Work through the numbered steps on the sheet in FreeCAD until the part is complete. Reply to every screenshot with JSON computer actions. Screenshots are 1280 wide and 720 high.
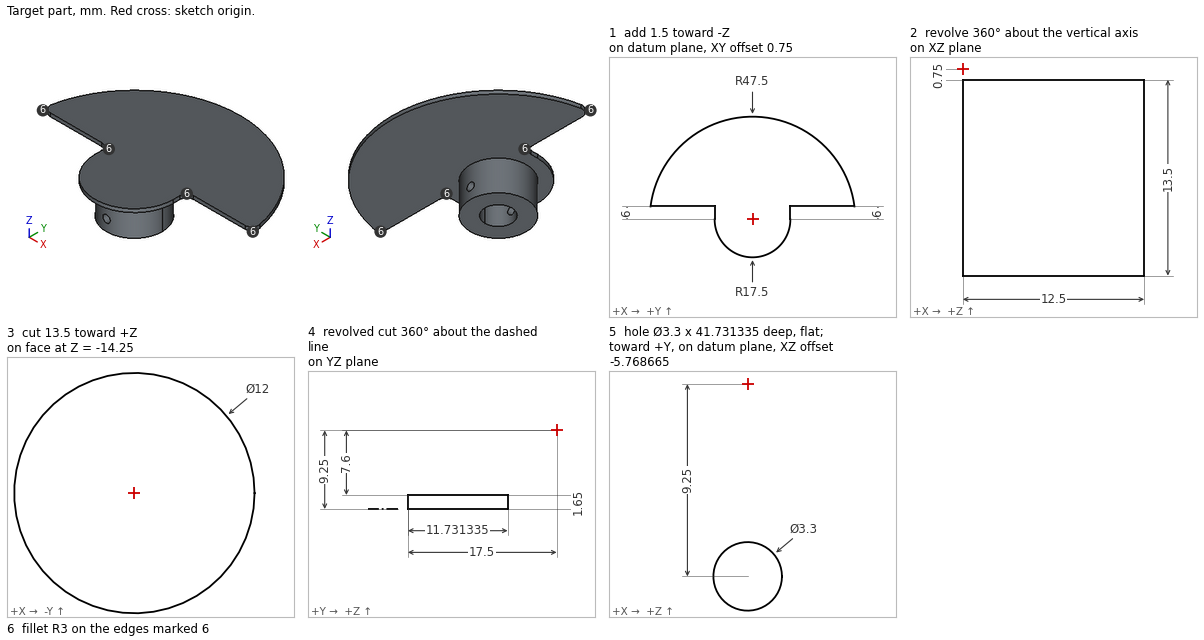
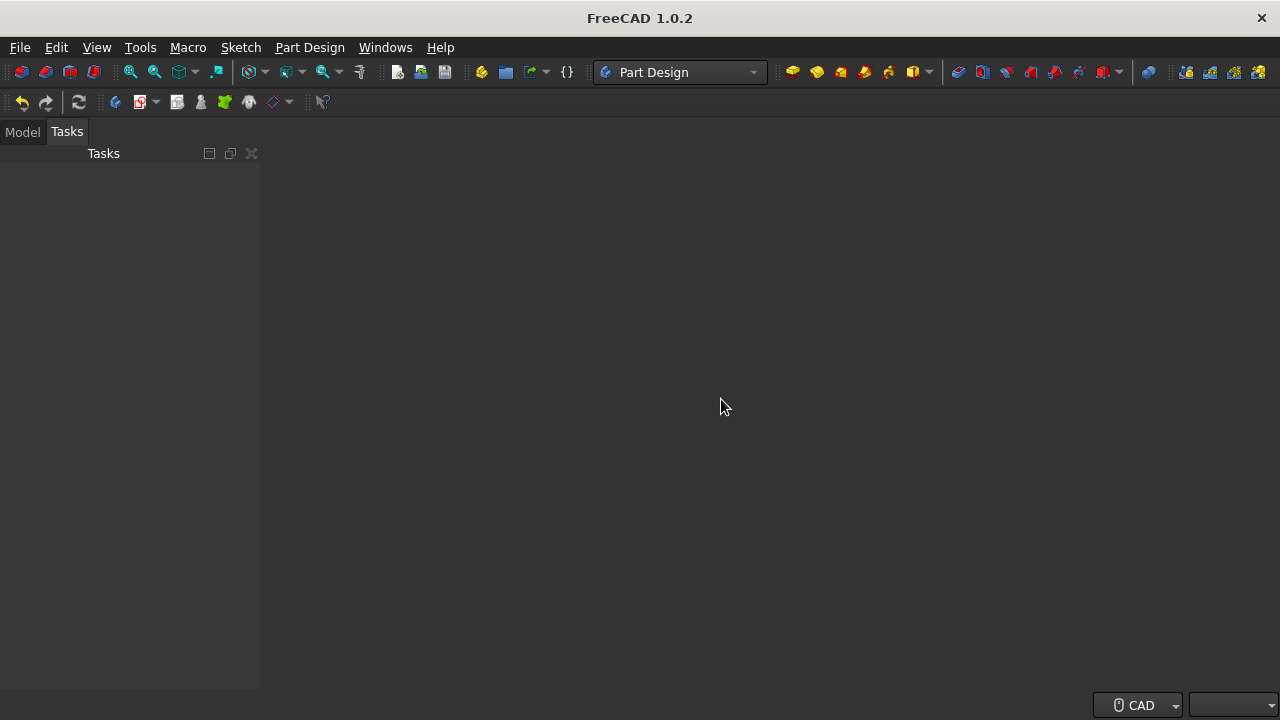
{"action": "left_click", "coordinate": [398, 72]}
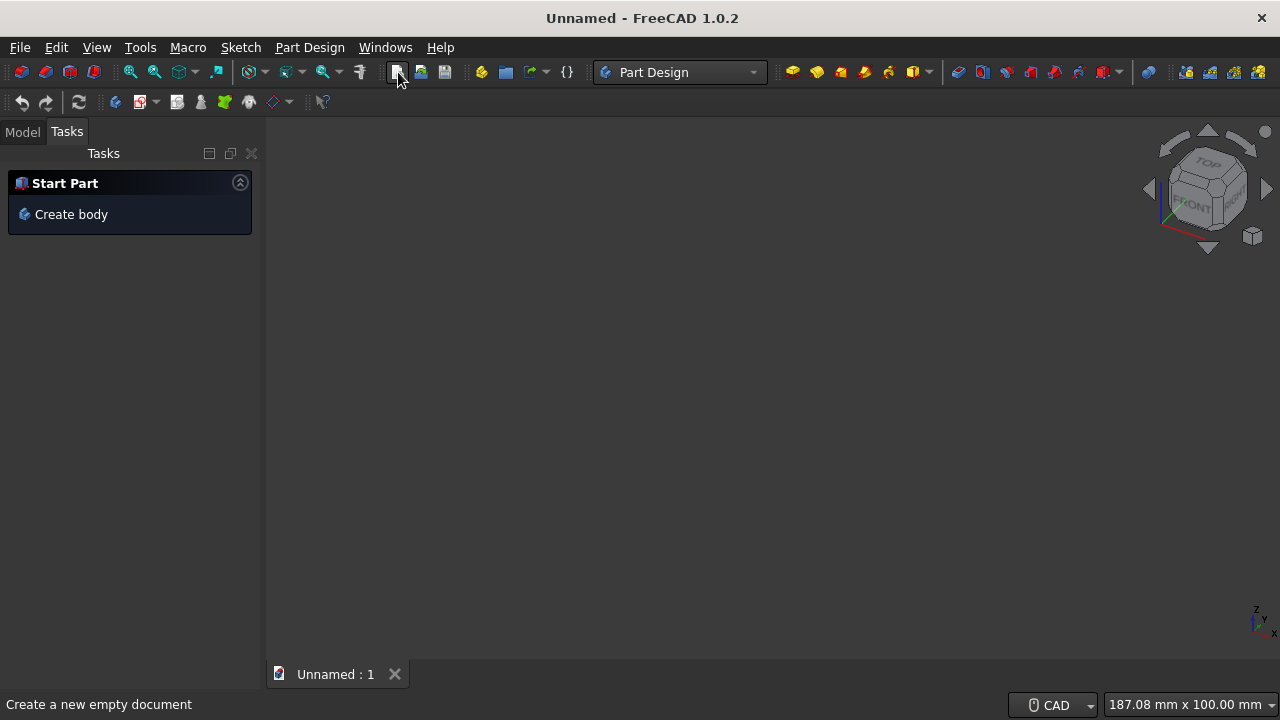
{"action": "left_click", "coordinate": [116, 102]}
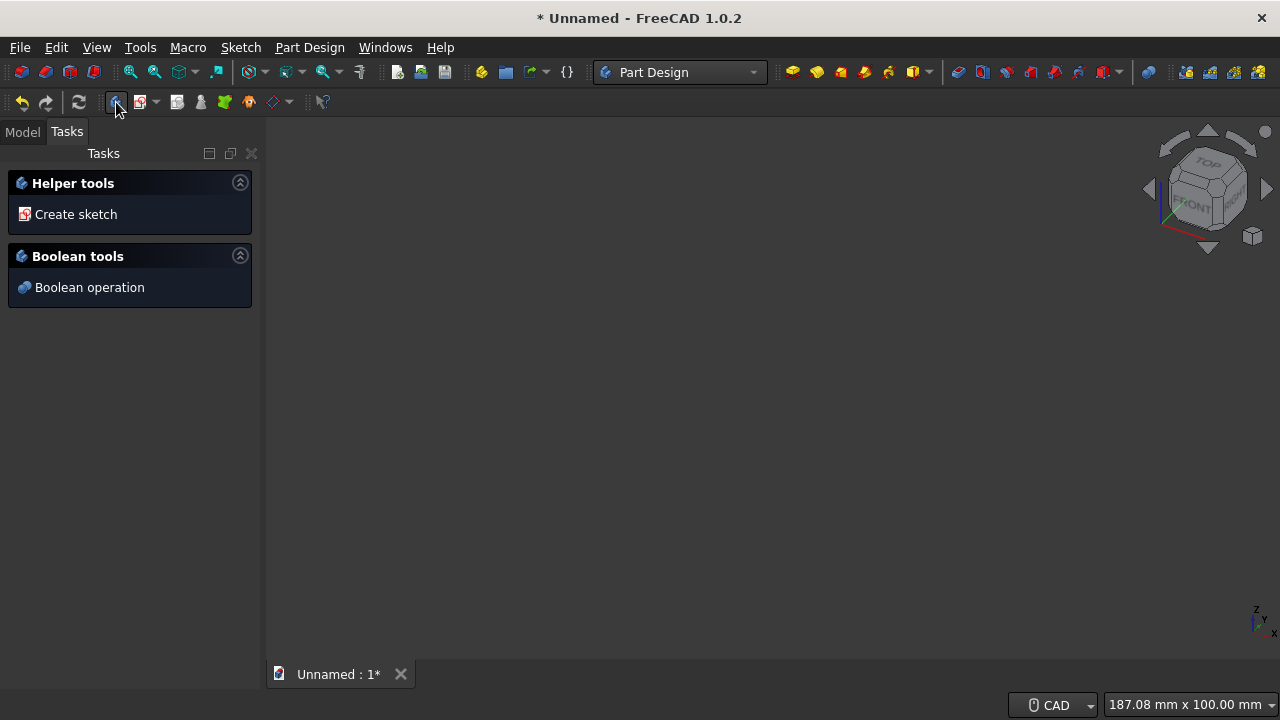
{"action": "left_click", "coordinate": [23, 131]}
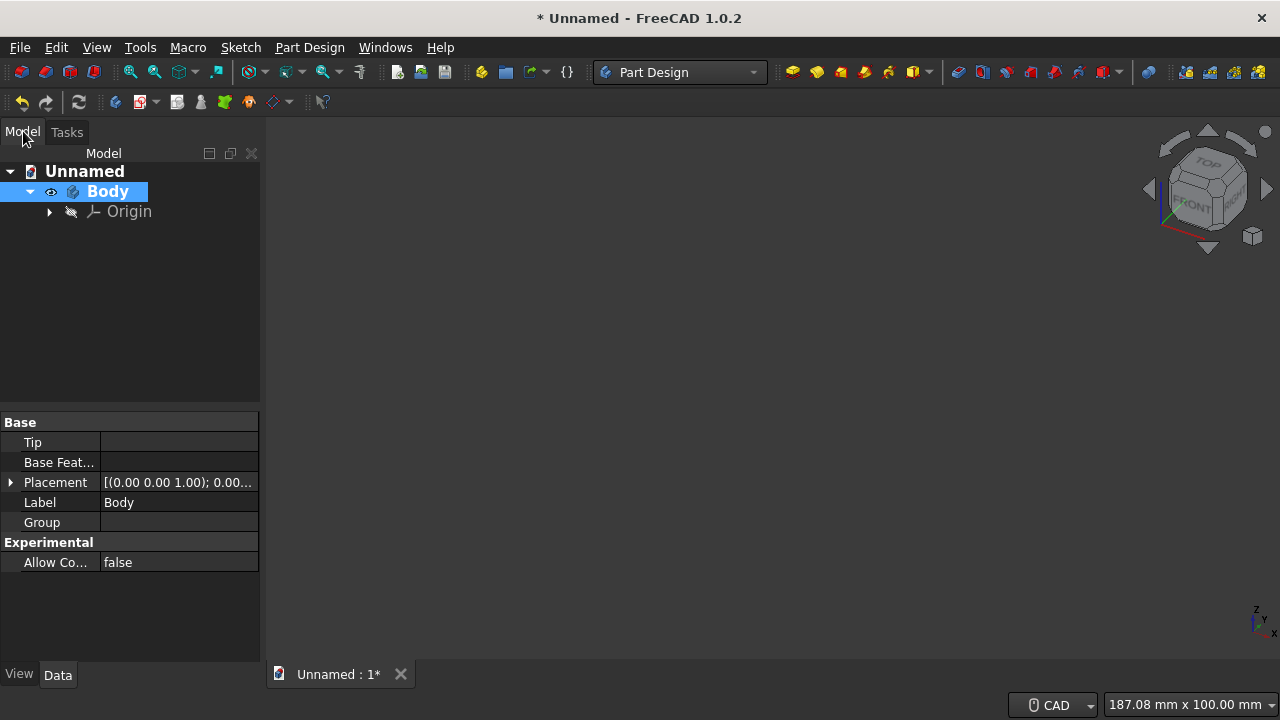
{"action": "left_click", "coordinate": [50, 212]}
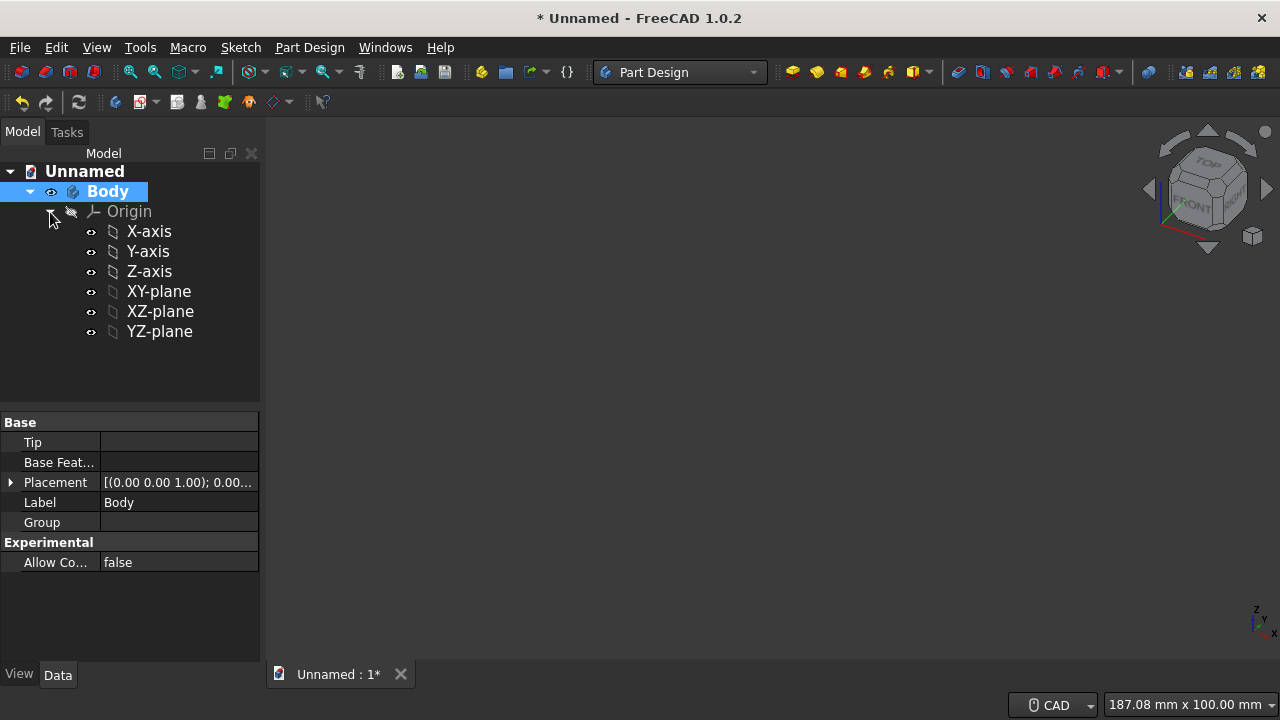
{"action": "left_click", "coordinate": [136, 292]}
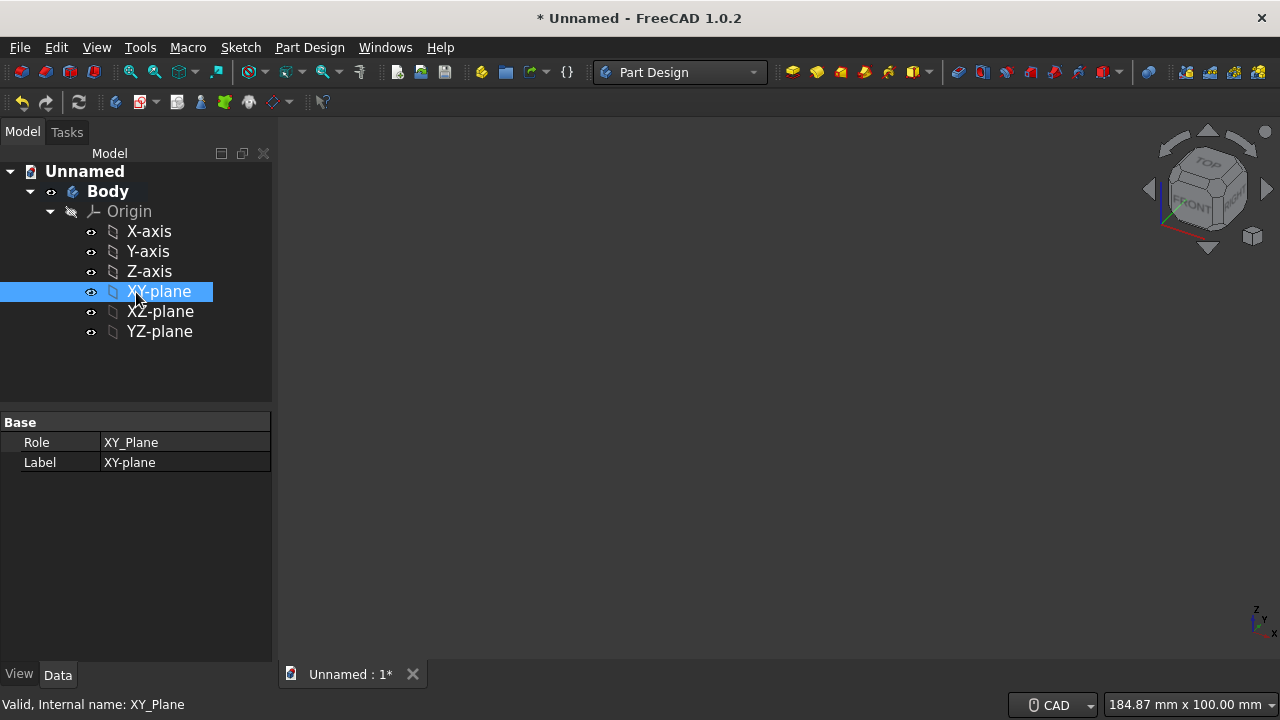
{"action": "left_click", "coordinate": [274, 102]}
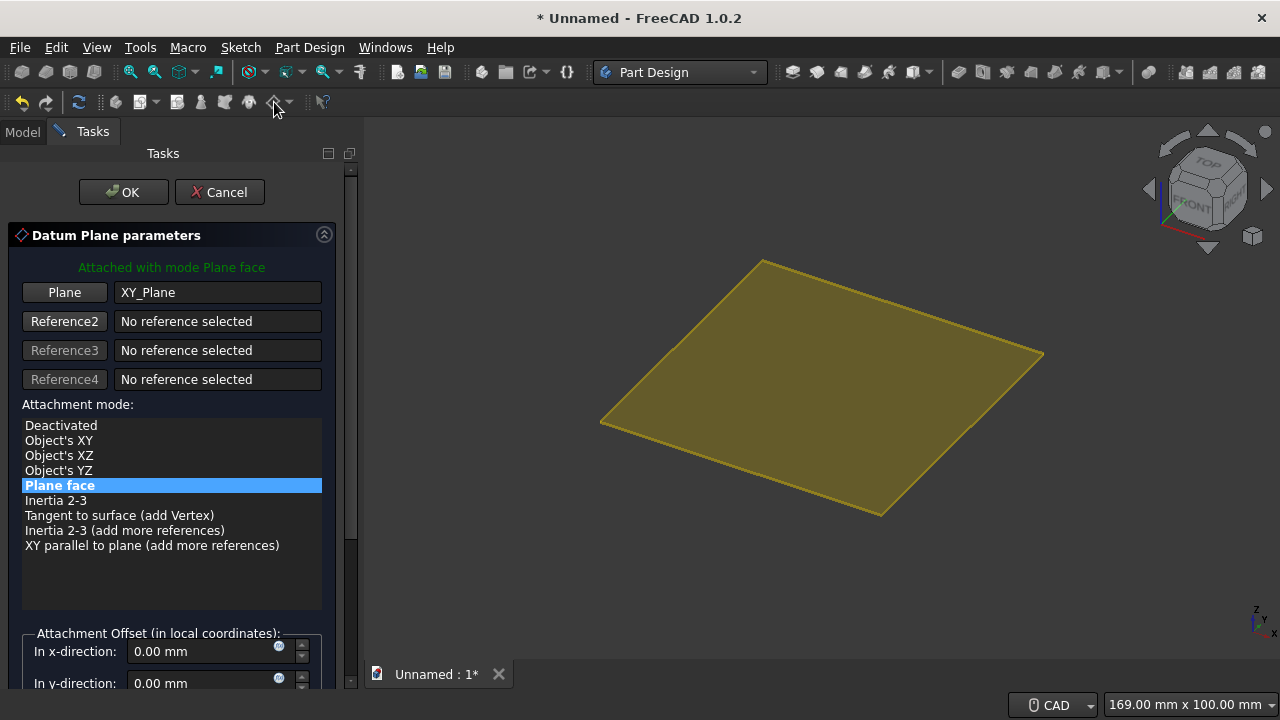
{"action": "scroll", "coordinate": [351, 426], "scroll_direction": "down", "scroll_amount": 2}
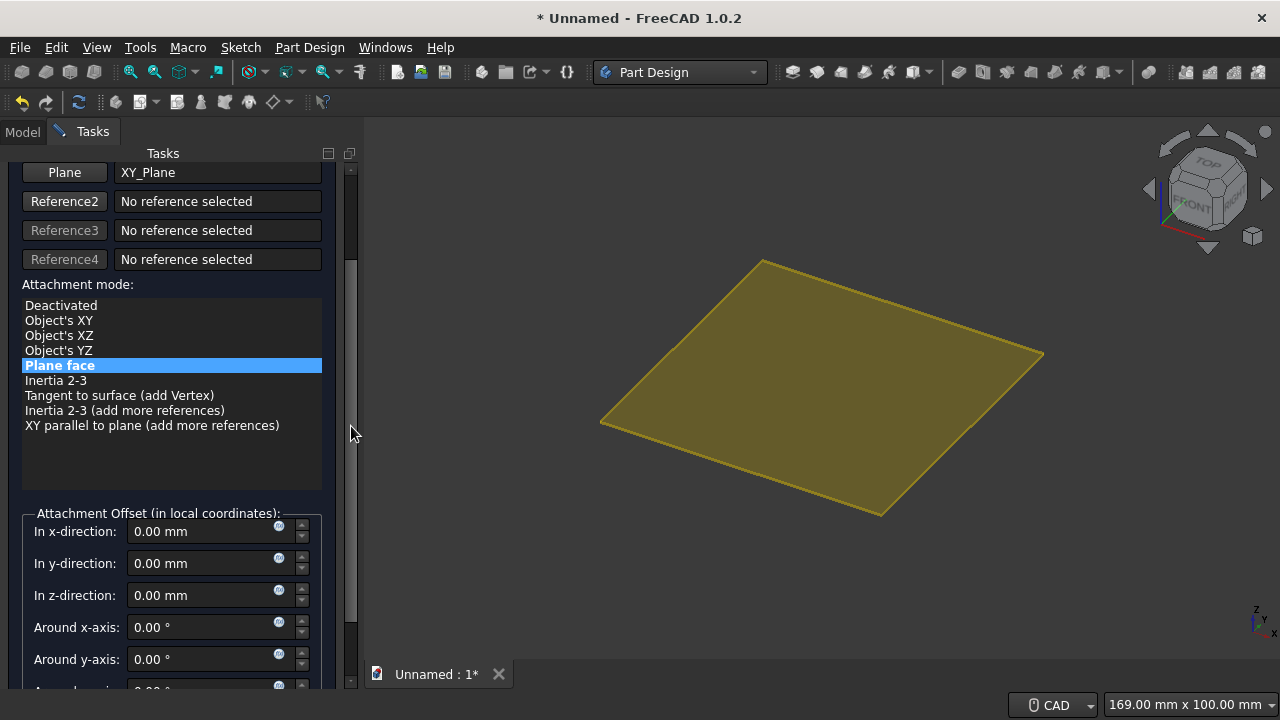
{"action": "triple_click", "coordinate": [210, 595]}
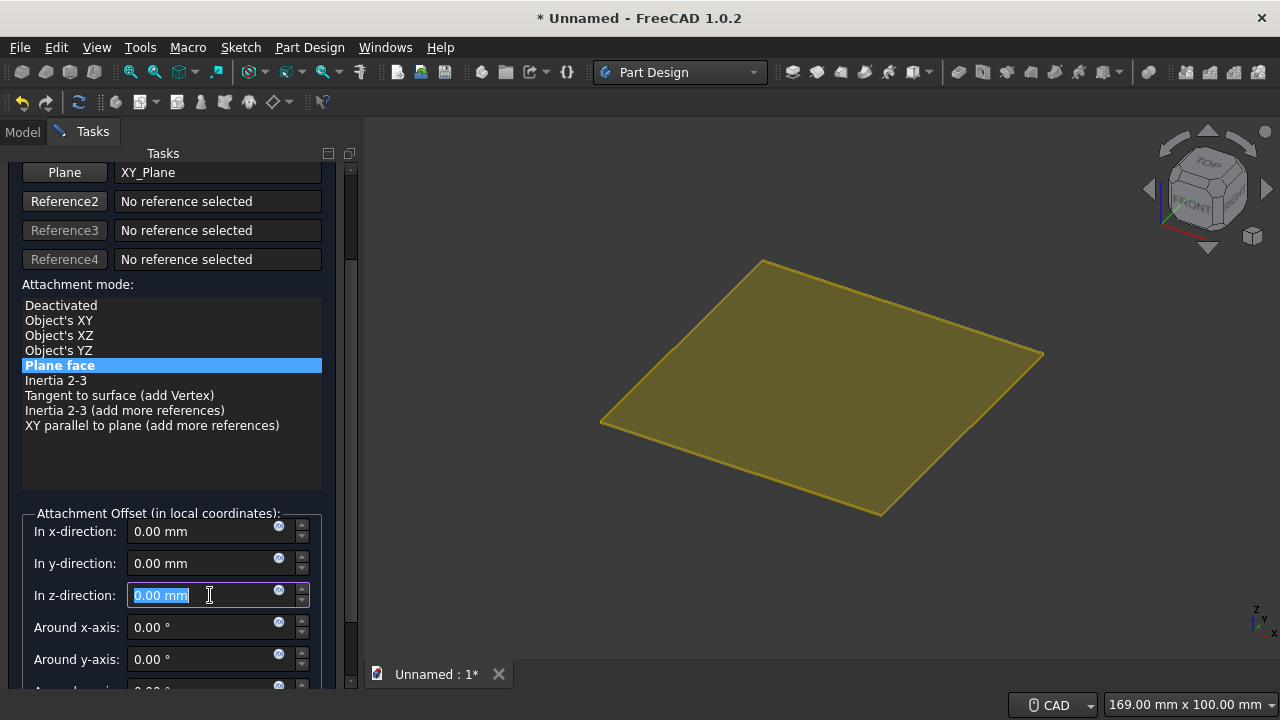
{"action": "type", "text": "0.75"}
{"action": "key", "text": "Tab"}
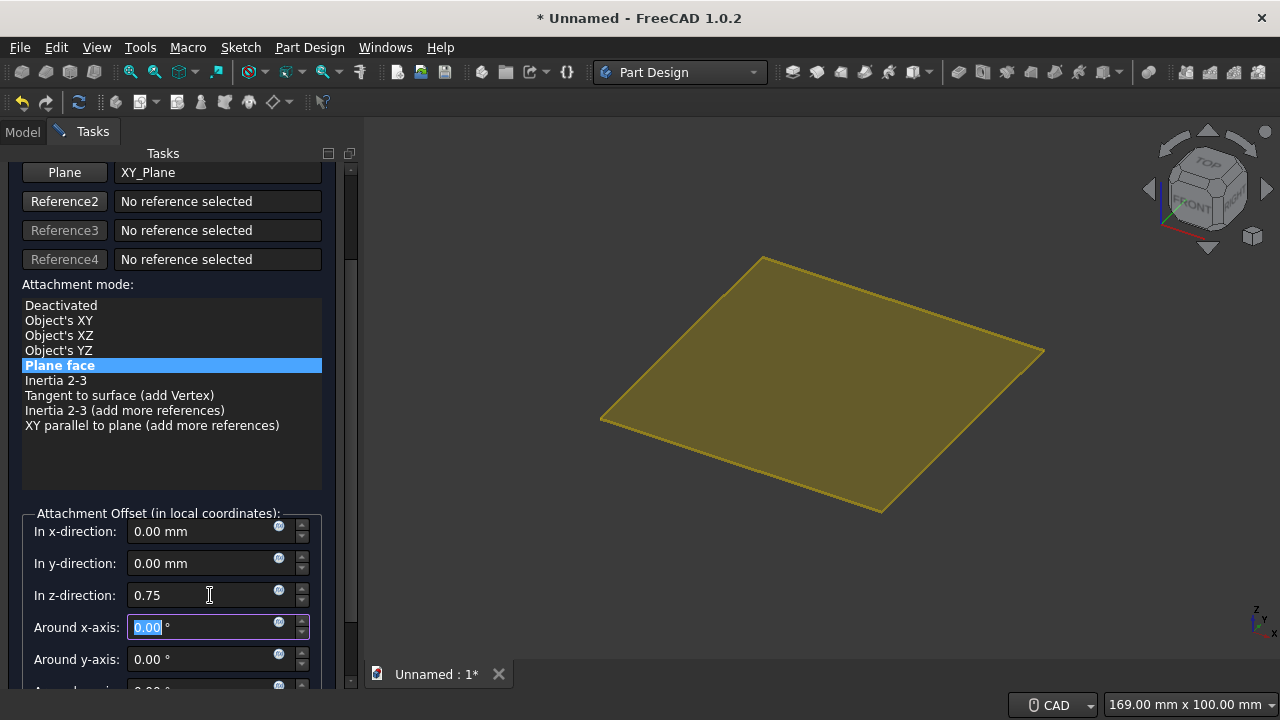
{"action": "scroll", "coordinate": [351, 426], "scroll_direction": "up", "scroll_amount": 3}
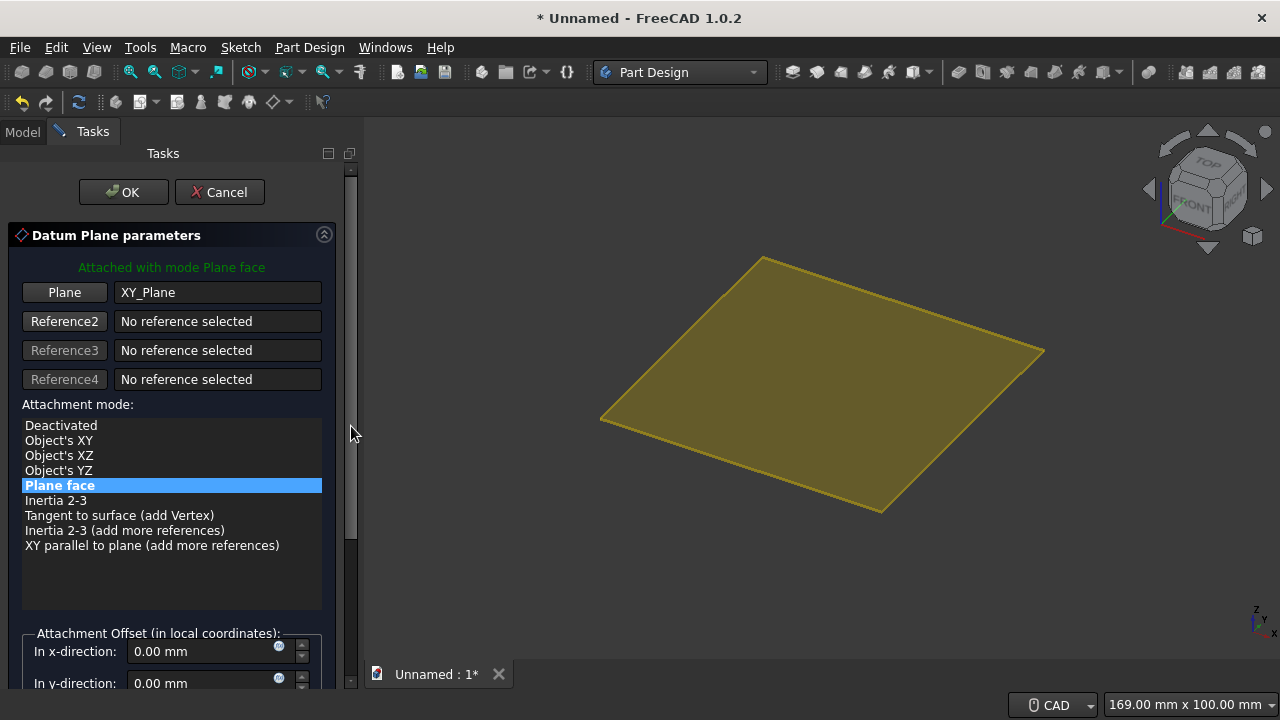
{"action": "left_click", "coordinate": [124, 192]}